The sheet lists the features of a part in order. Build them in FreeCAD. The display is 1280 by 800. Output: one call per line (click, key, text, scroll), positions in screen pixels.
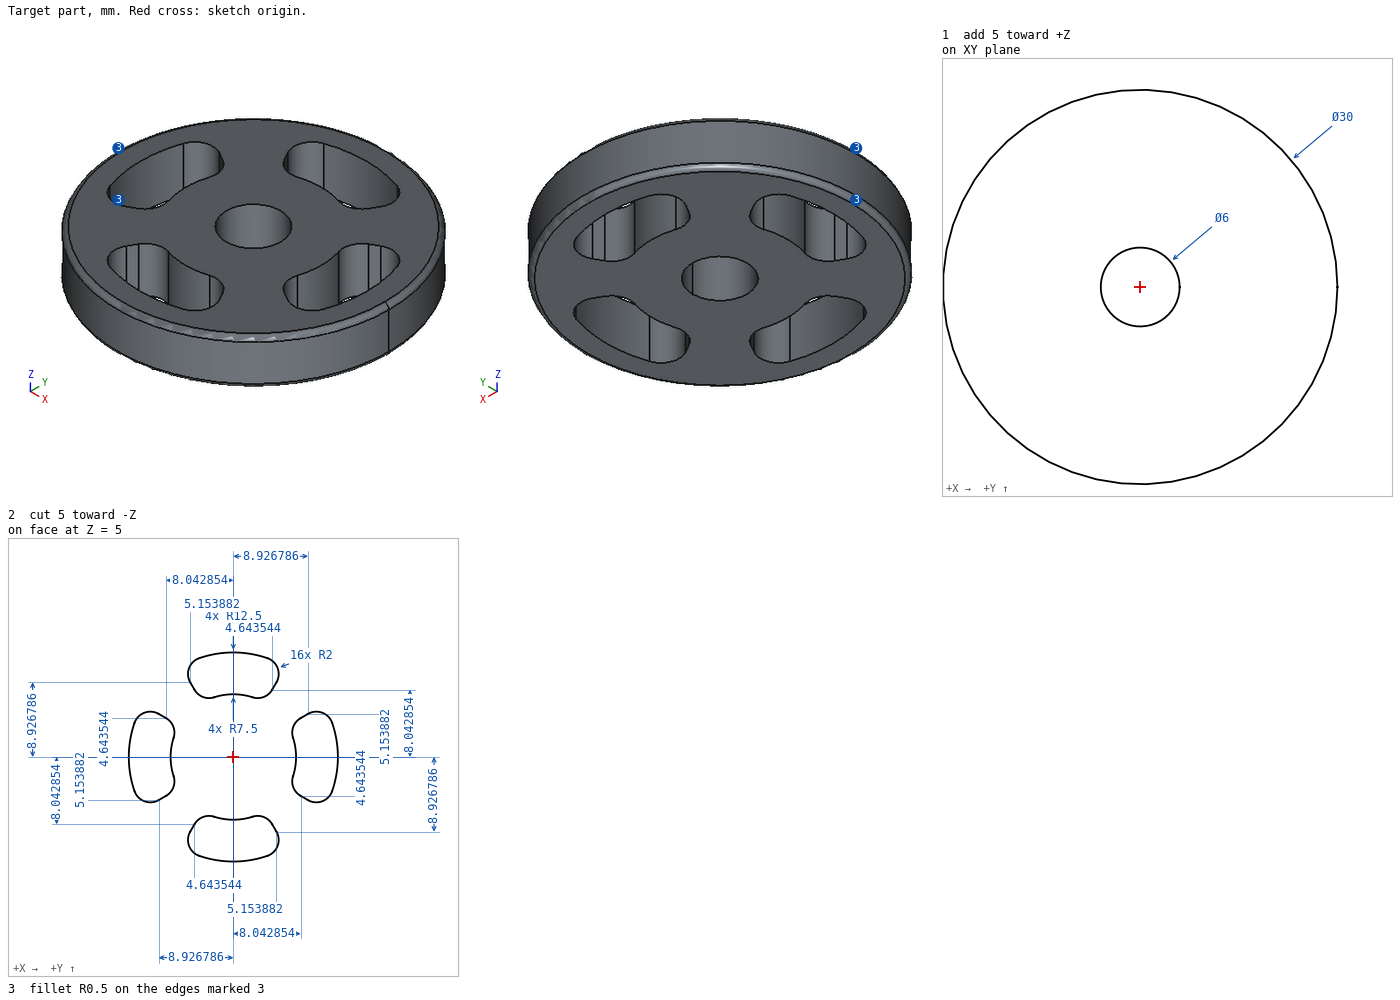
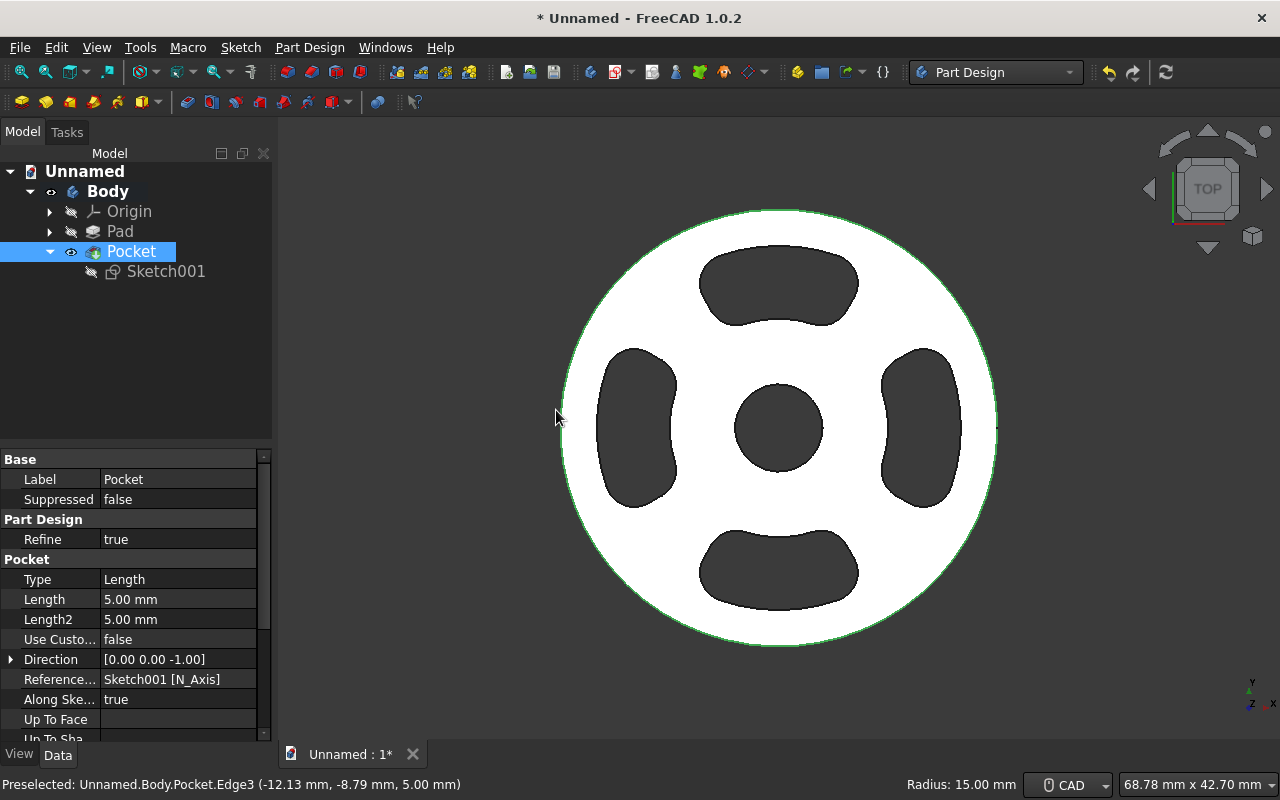
key(1)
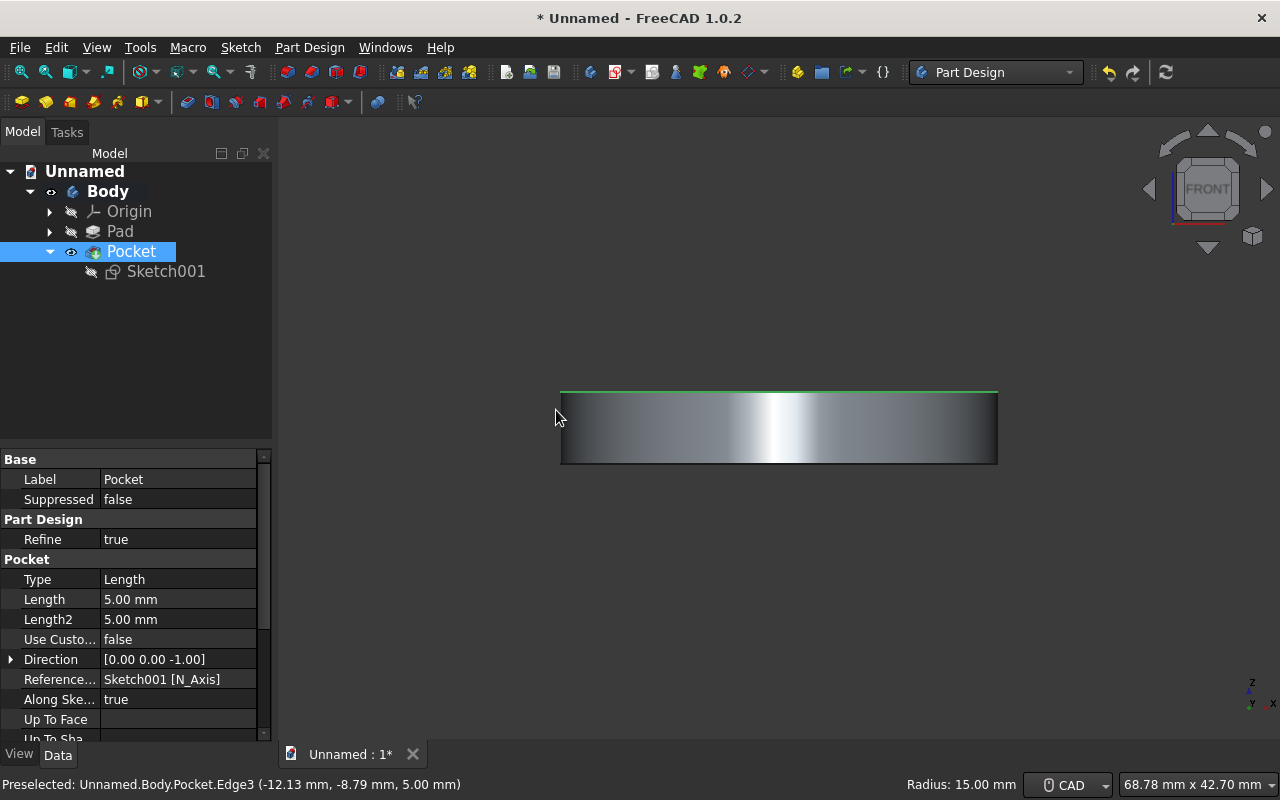
click(22, 72)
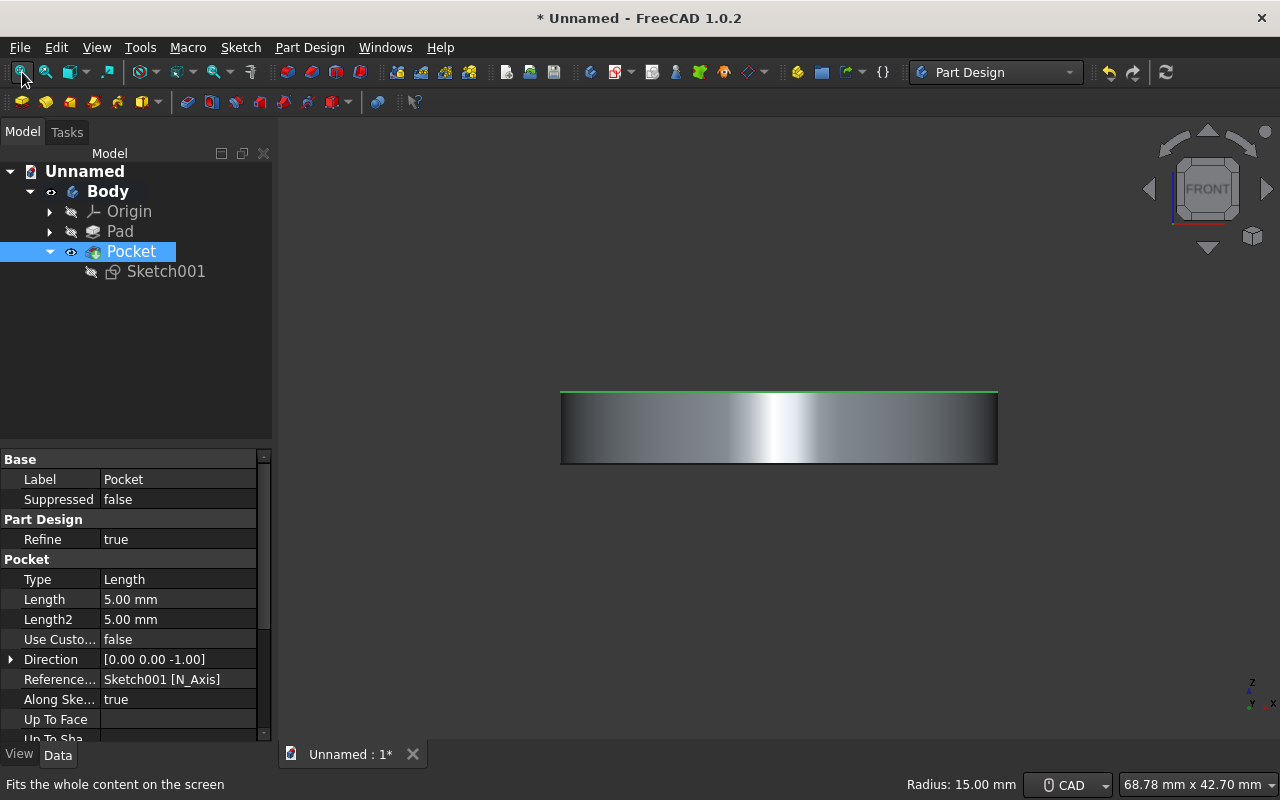
click(602, 463, ctrl)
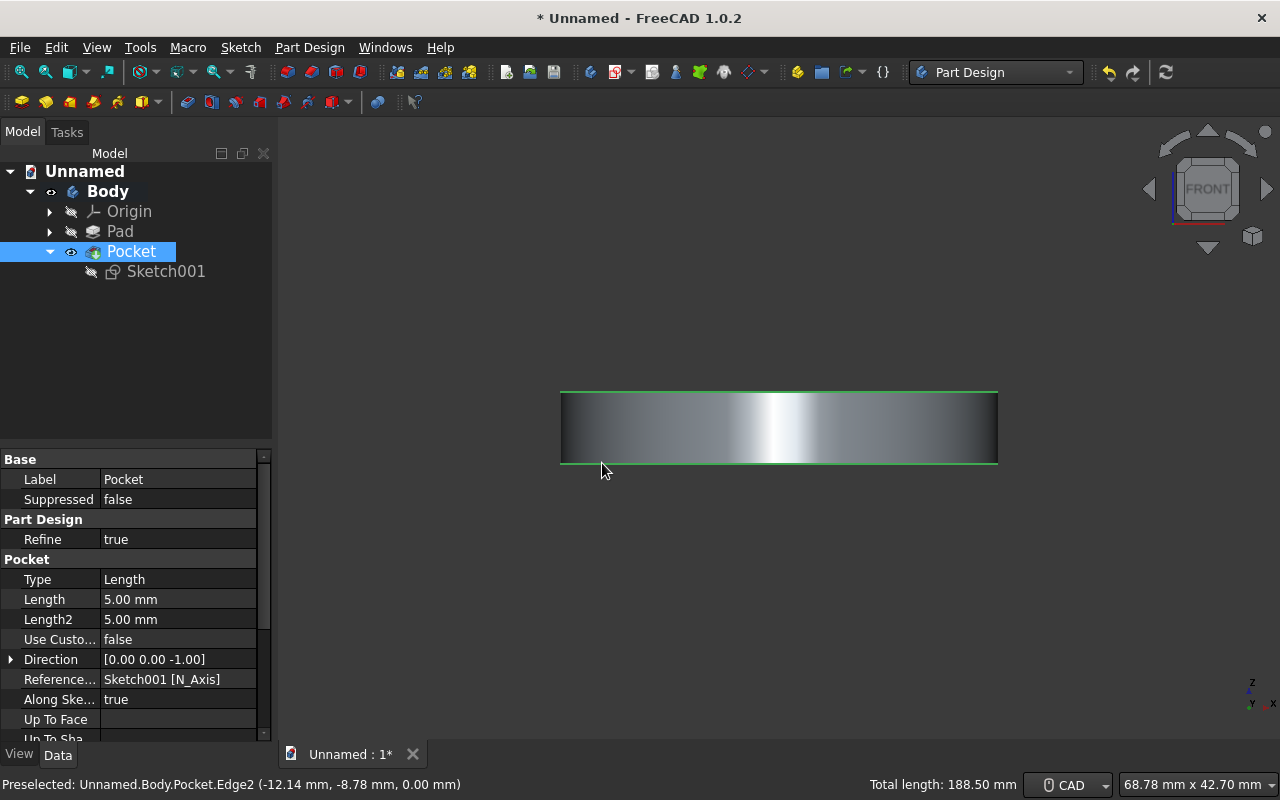
click(288, 72)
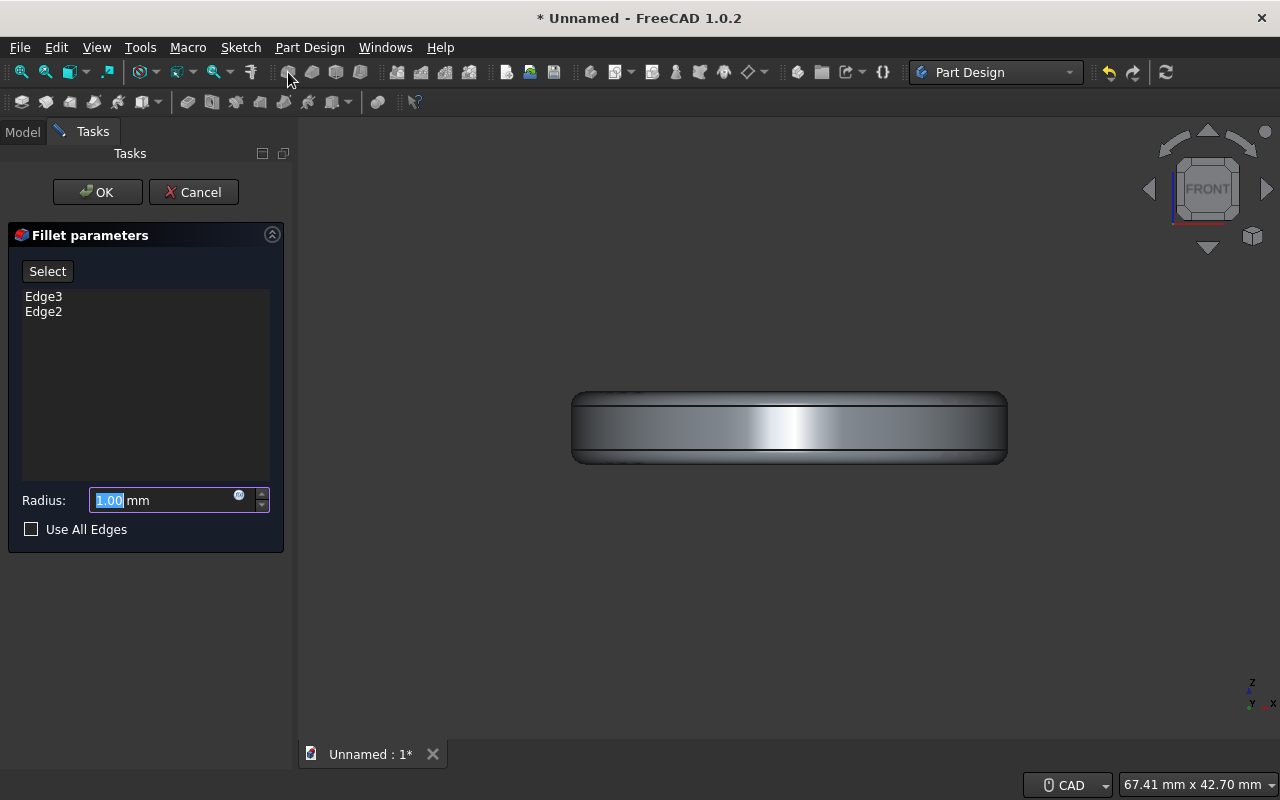
text(0.5)
key(Tab)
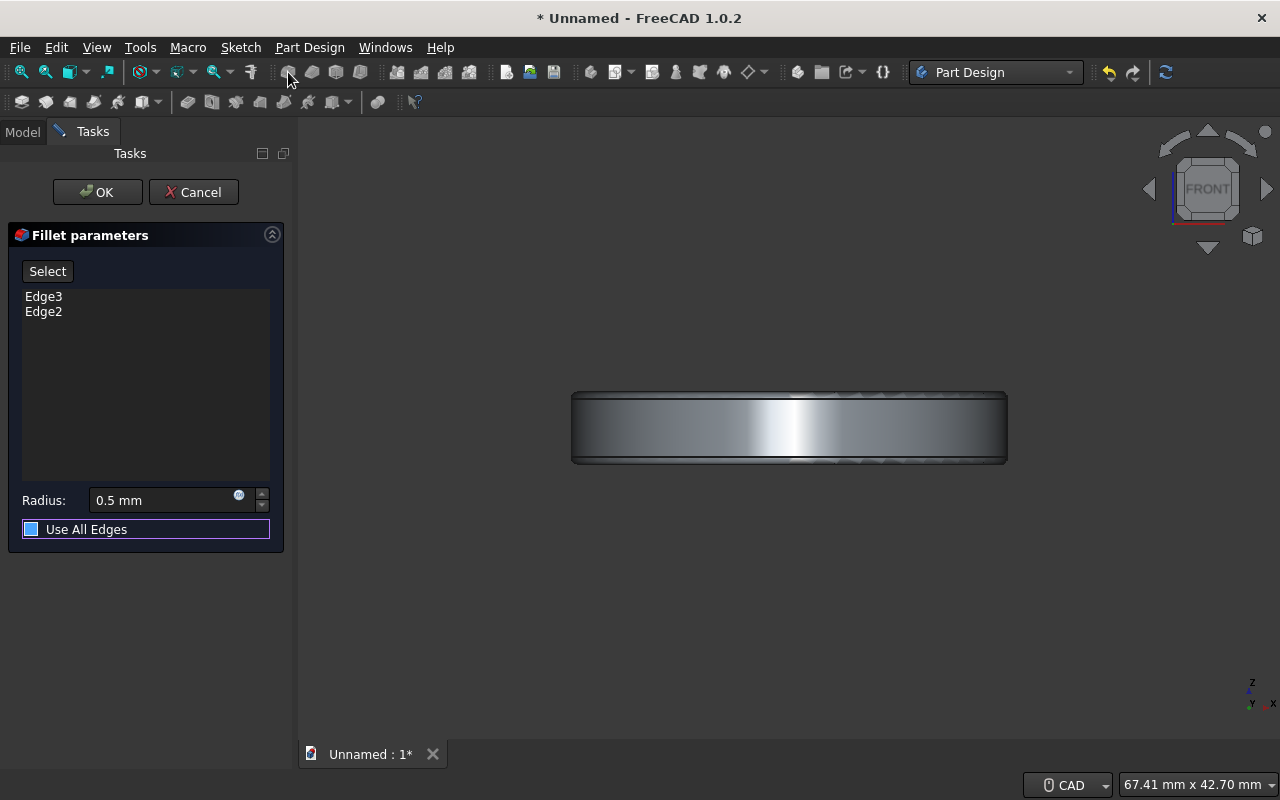
click(98, 192)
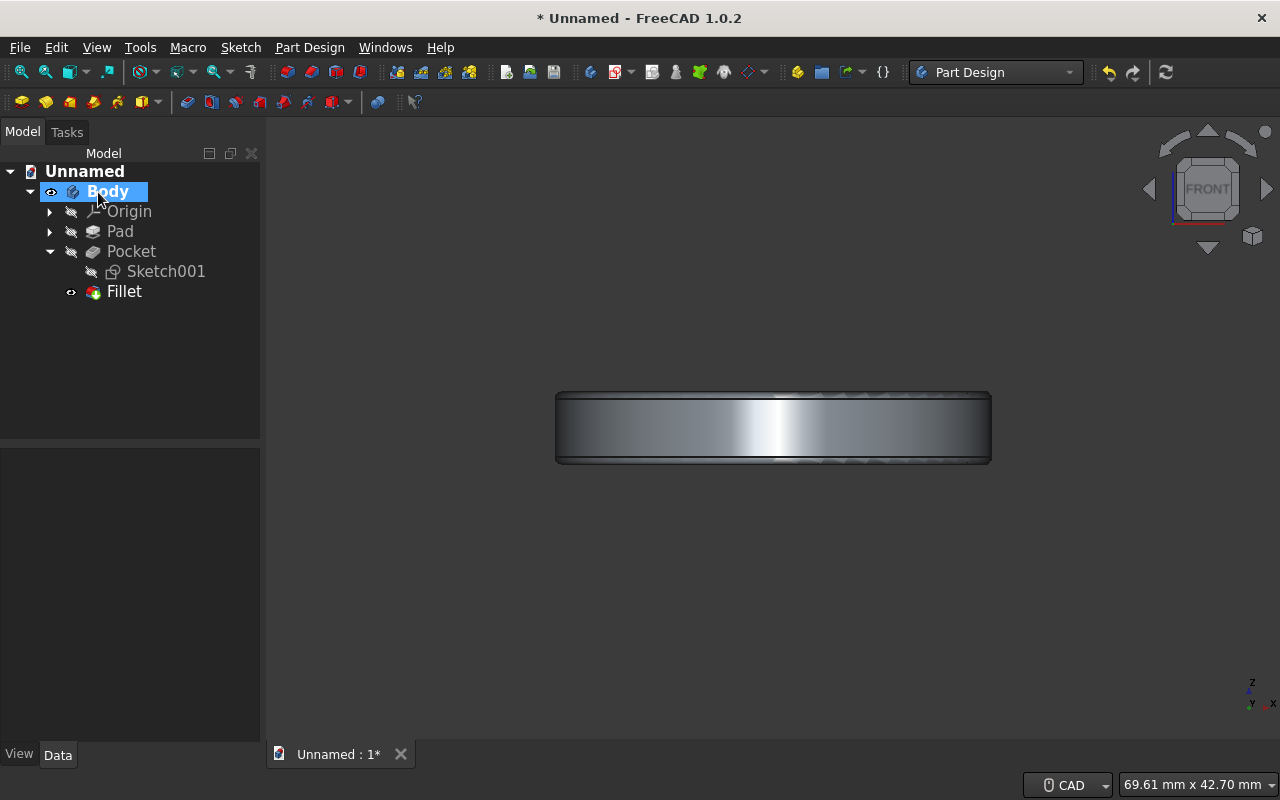
key(0)